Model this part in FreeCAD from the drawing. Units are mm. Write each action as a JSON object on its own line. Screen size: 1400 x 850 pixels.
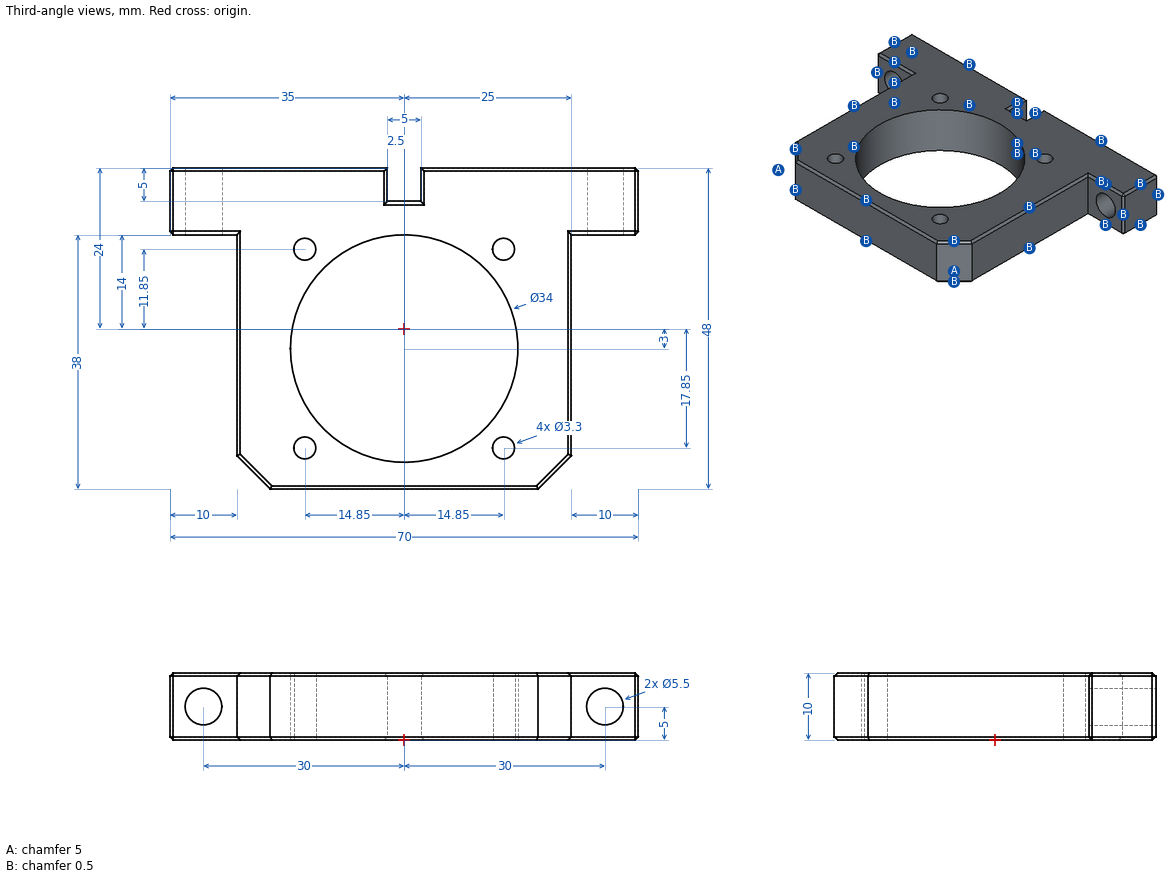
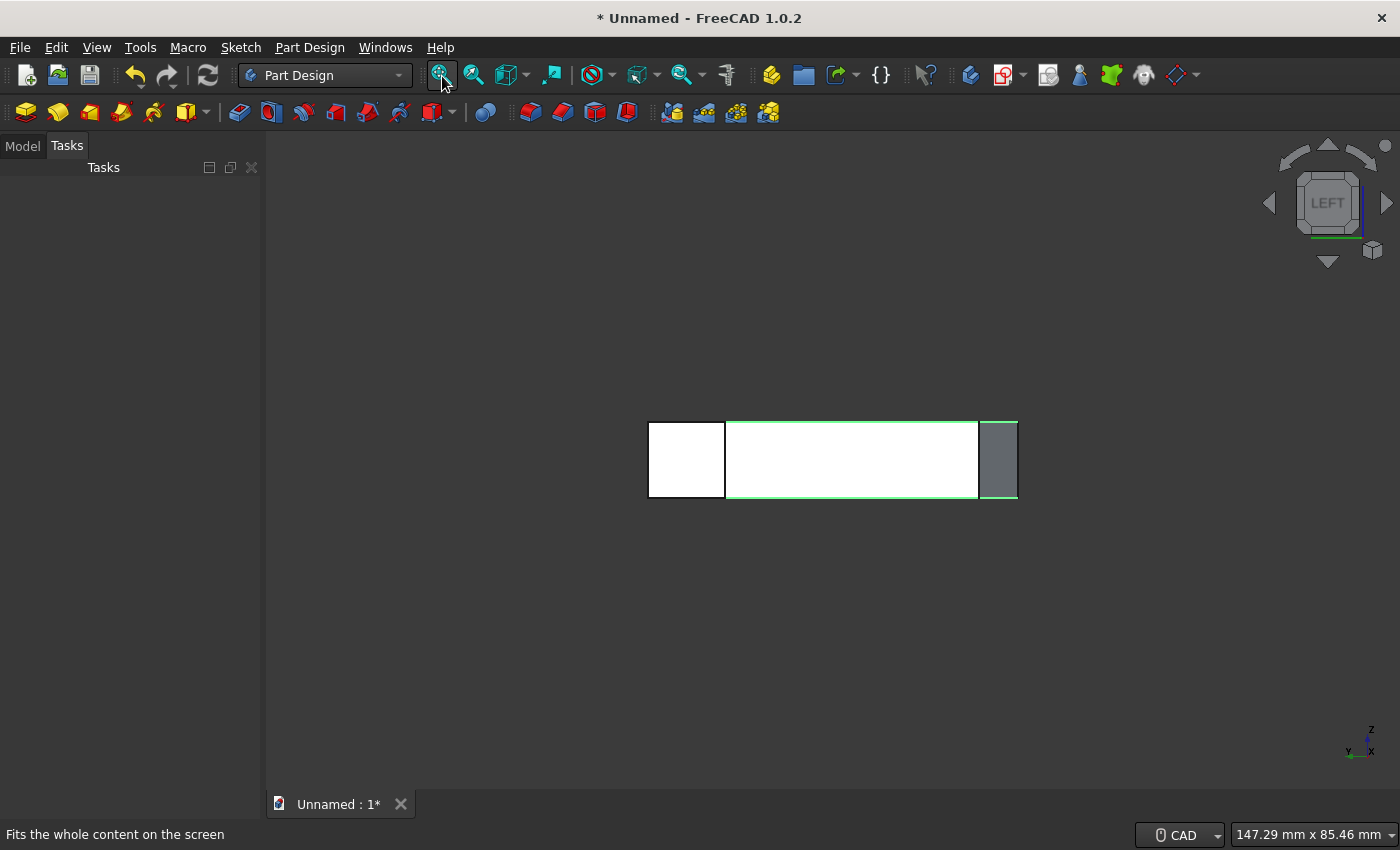
{"action": "left_click", "coordinate": [687, 459], "text": "ctrl"}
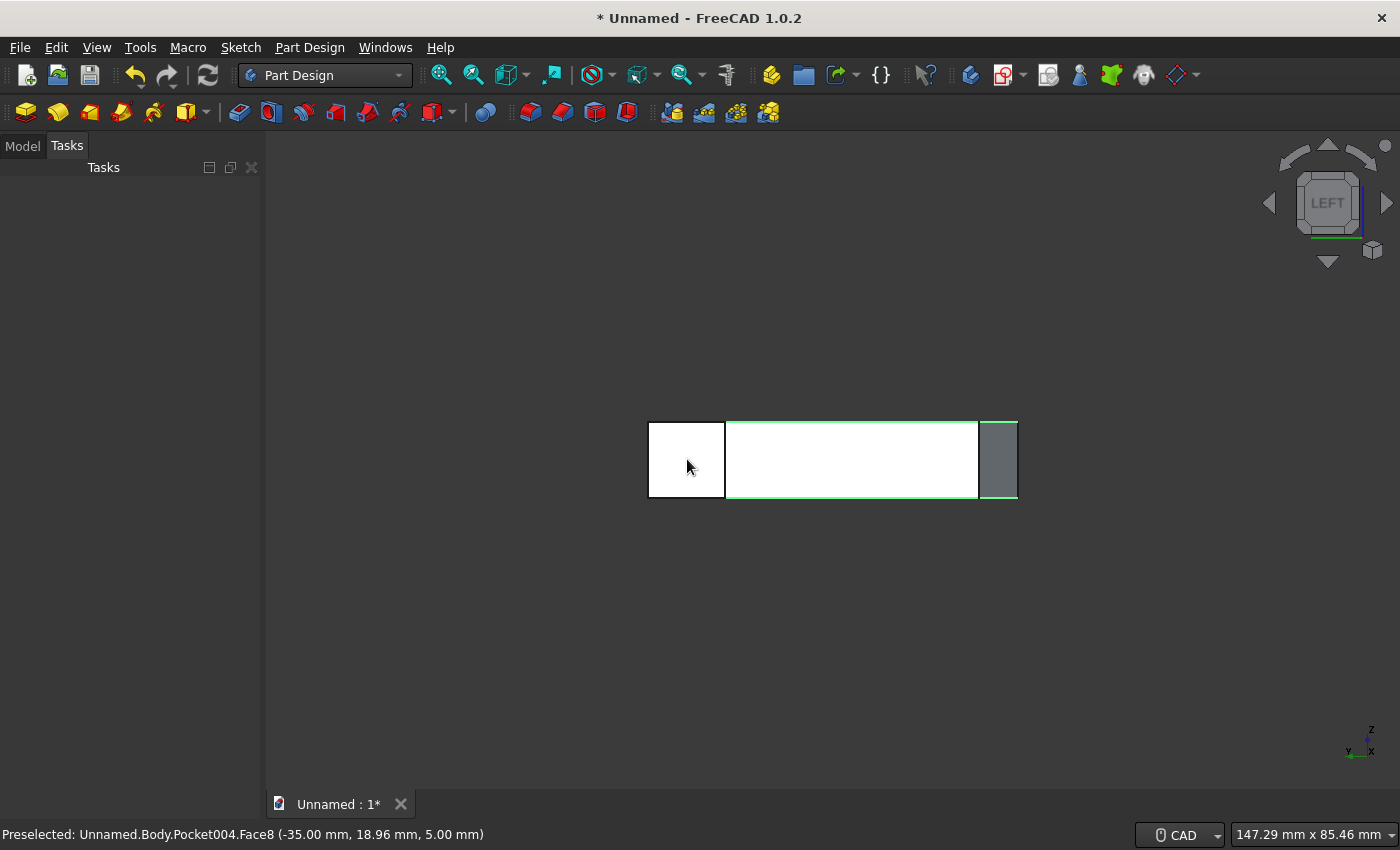
{"action": "left_click", "coordinate": [564, 112]}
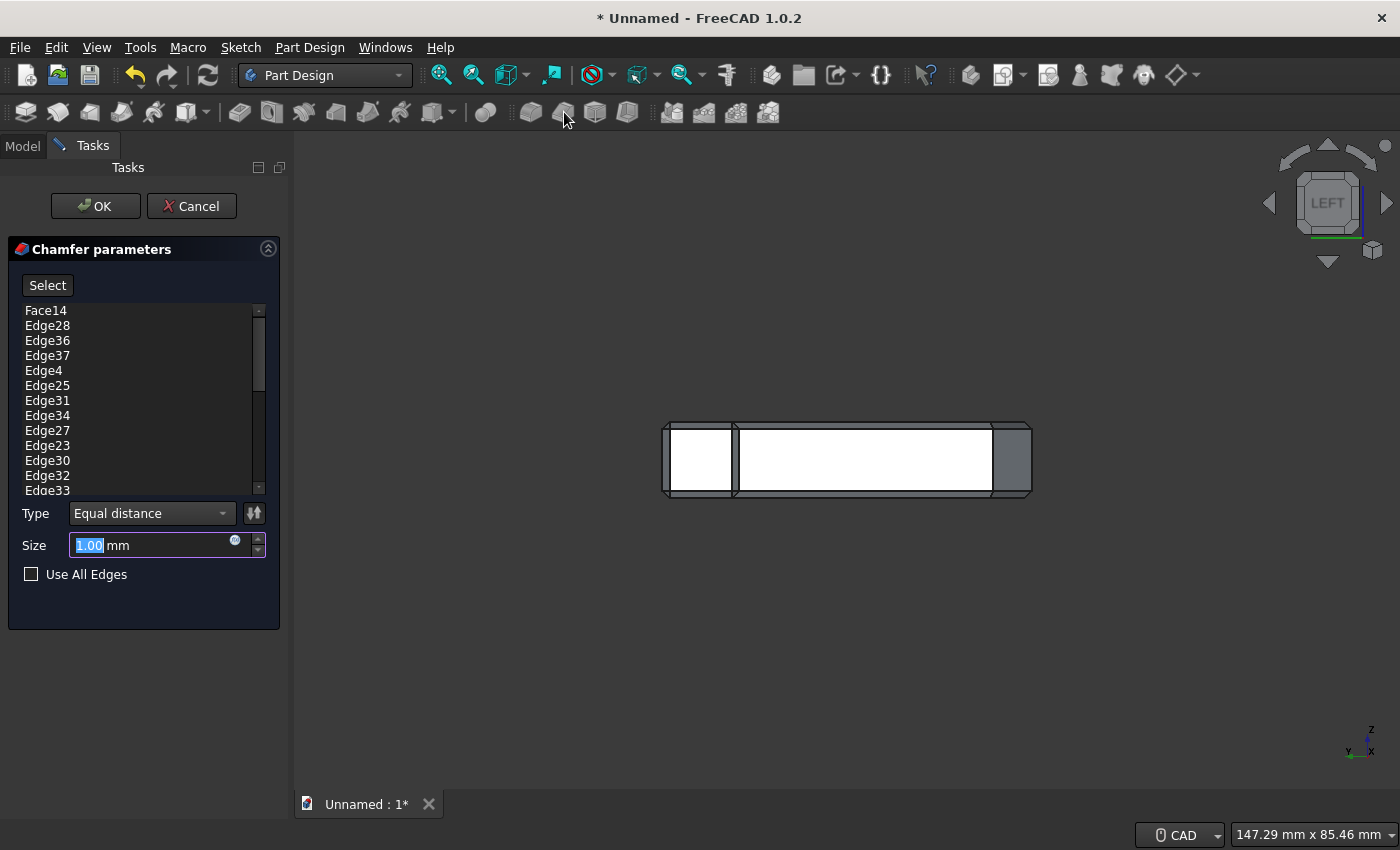
{"action": "type", "text": "0.5"}
{"action": "key", "text": "Tab"}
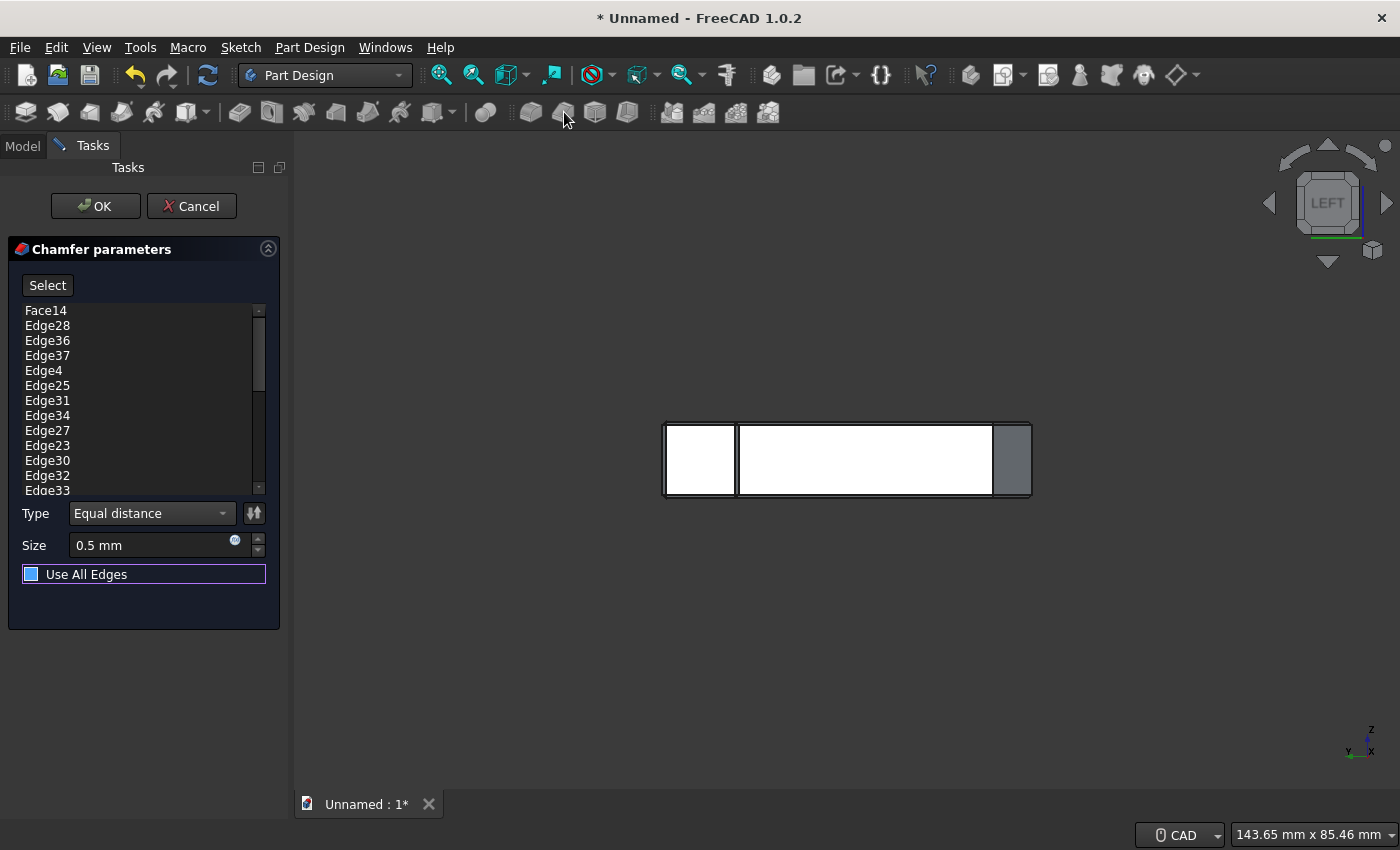
{"action": "left_click", "coordinate": [96, 206]}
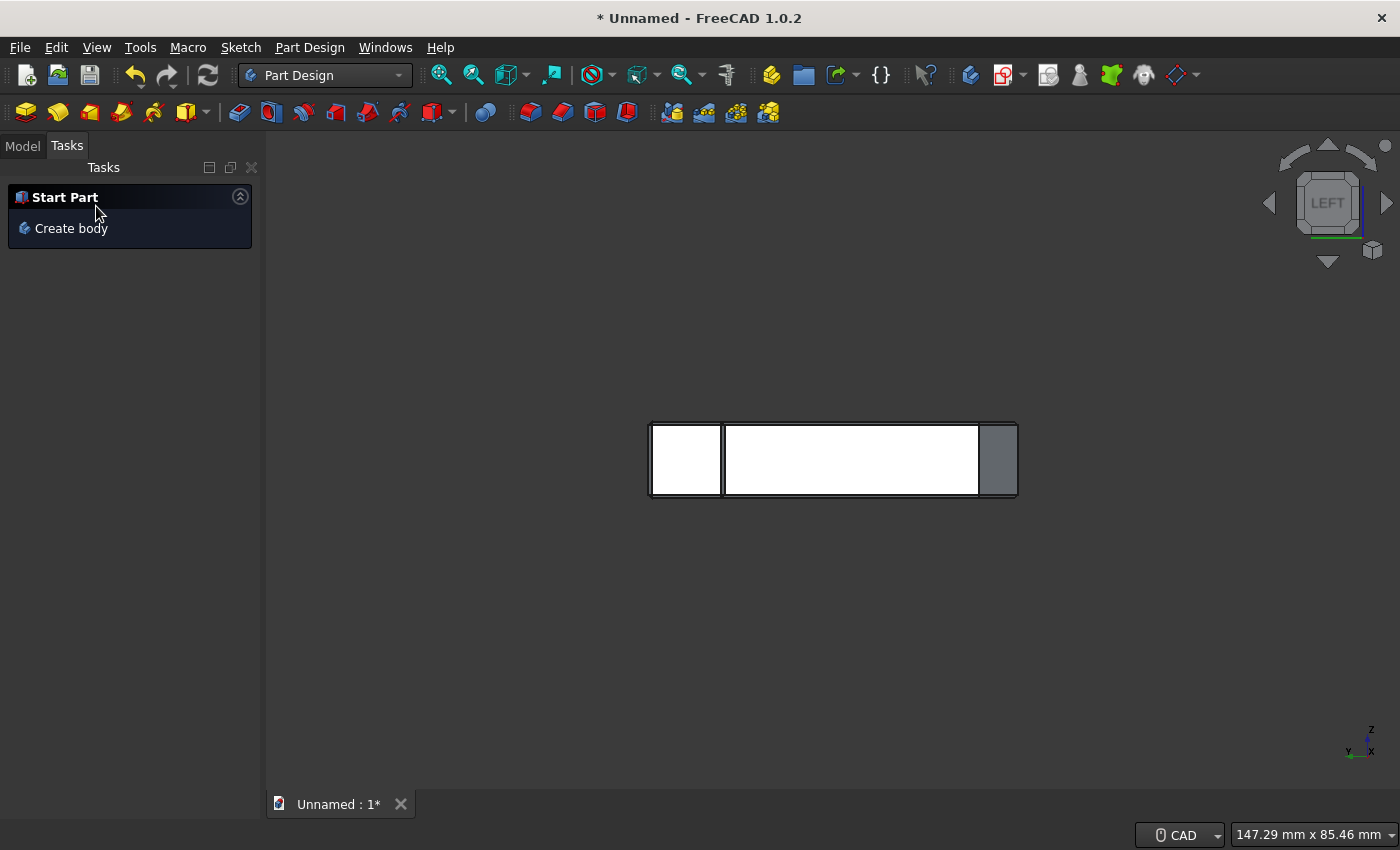
{"action": "key", "text": "0"}